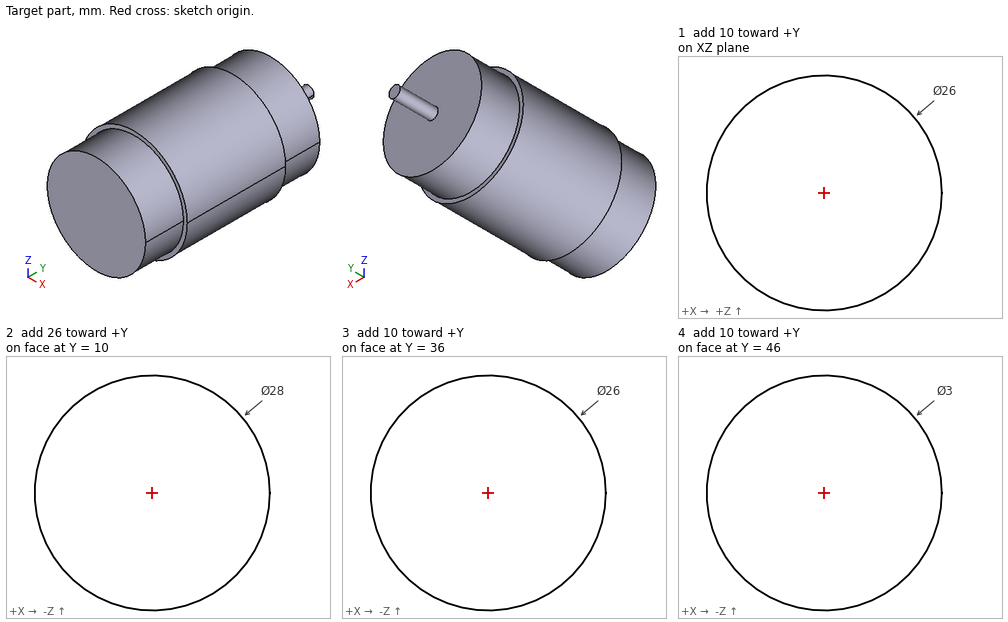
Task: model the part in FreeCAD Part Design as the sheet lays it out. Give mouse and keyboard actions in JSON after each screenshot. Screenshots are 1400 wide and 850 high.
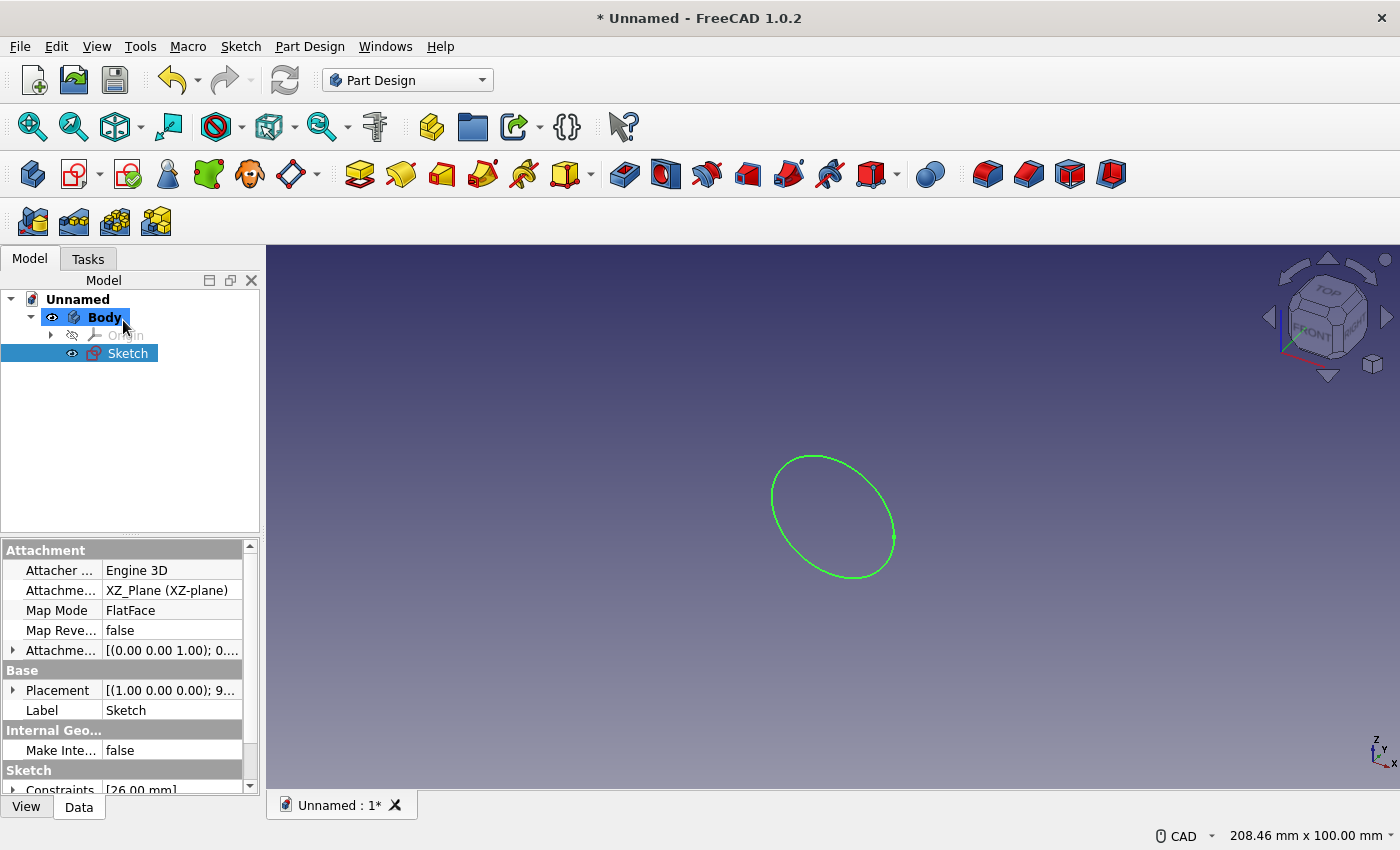
{"action": "left_click", "coordinate": [360, 174]}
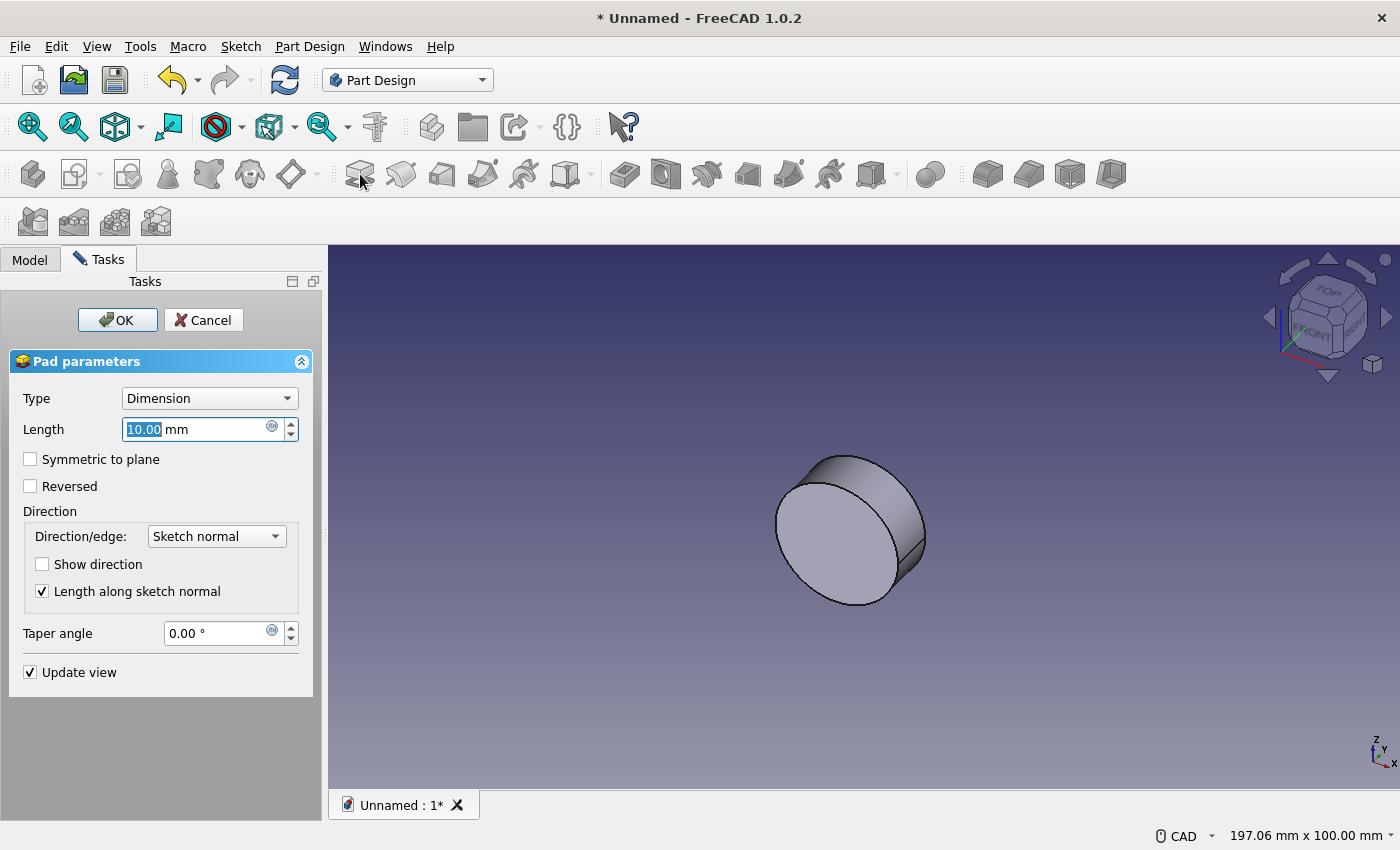
{"action": "type", "text": "10"}
{"action": "key", "text": "Tab"}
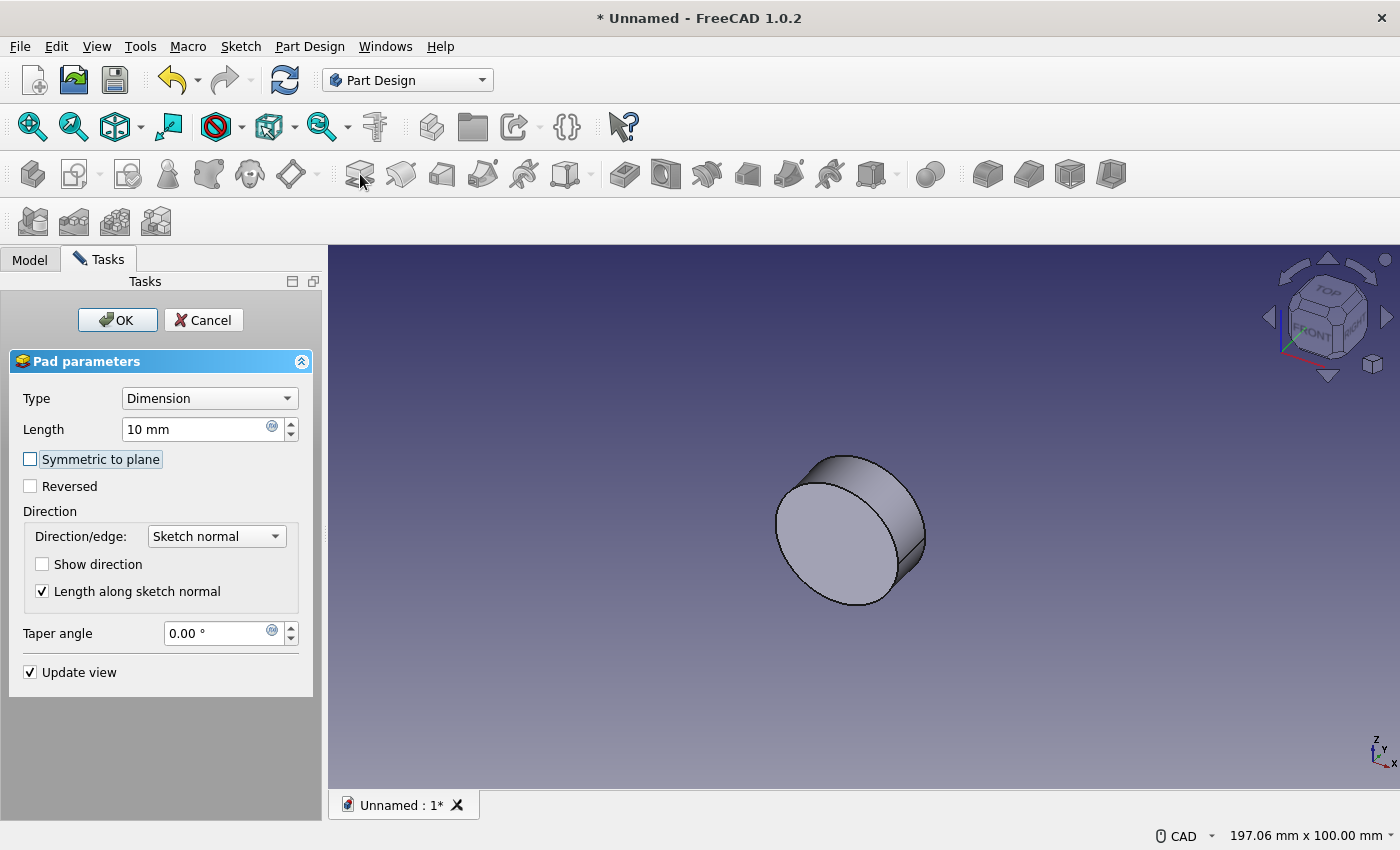
{"action": "left_click", "coordinate": [31, 486]}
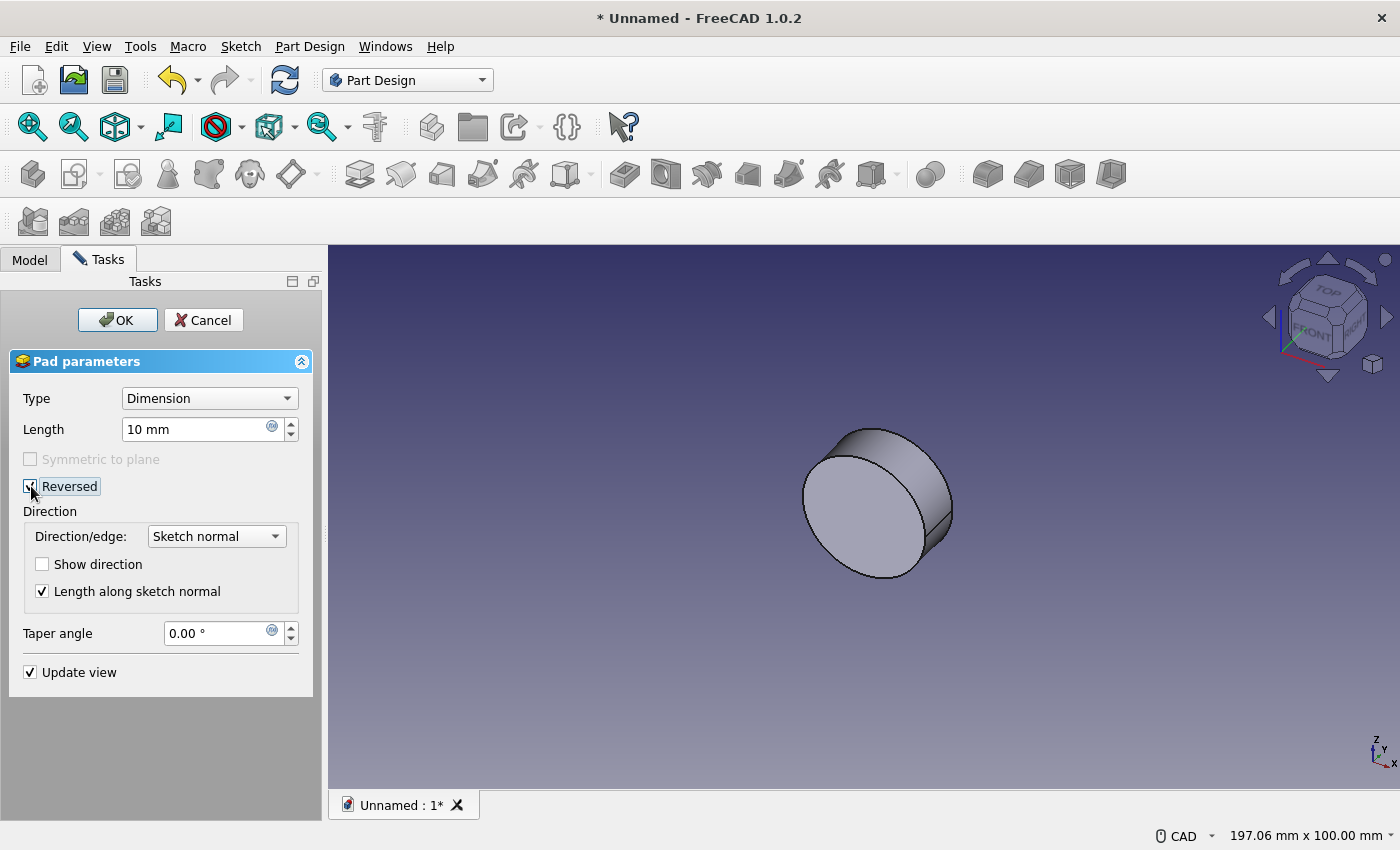
{"action": "left_click", "coordinate": [118, 320]}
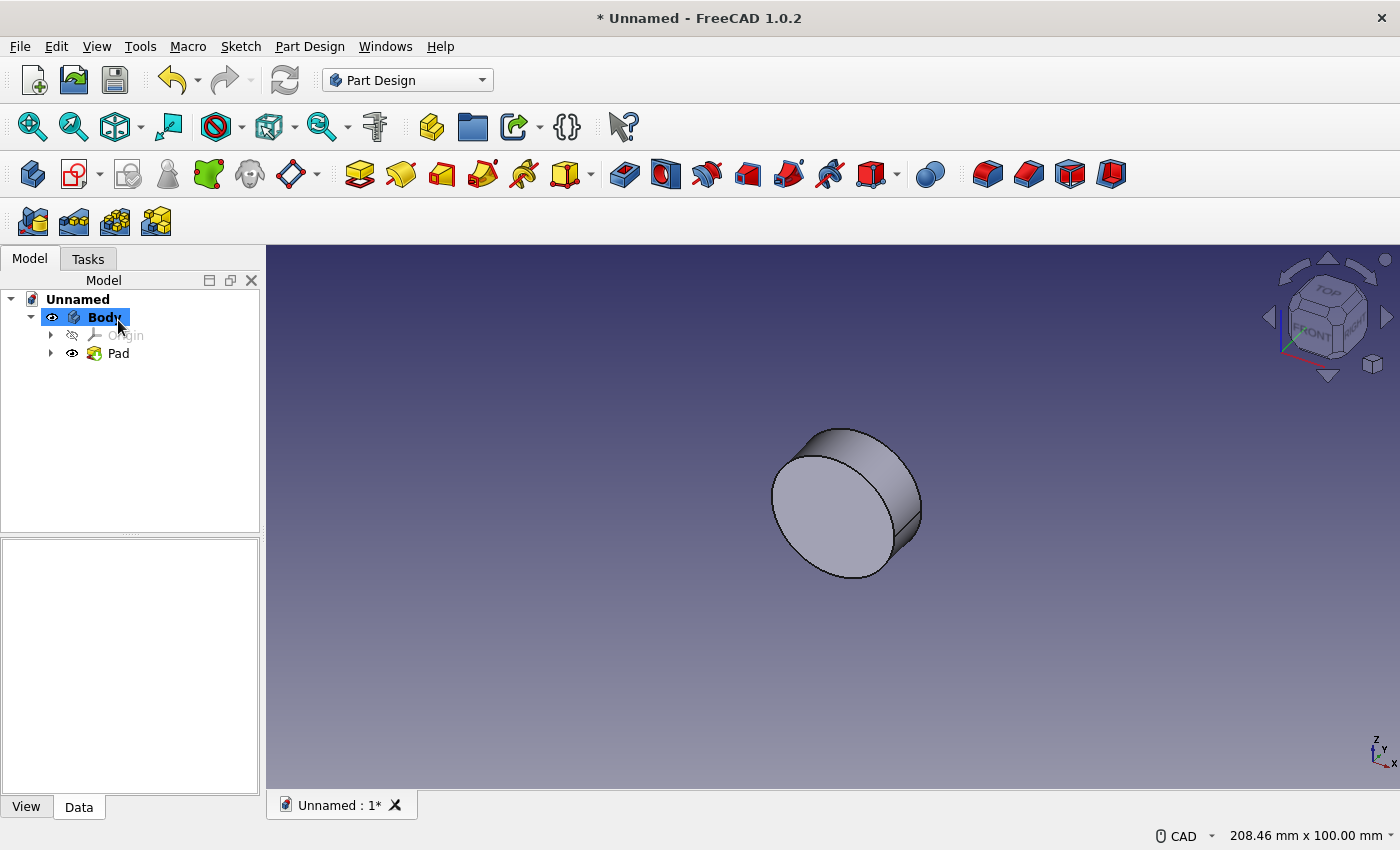
{"action": "left_click", "coordinate": [33, 128]}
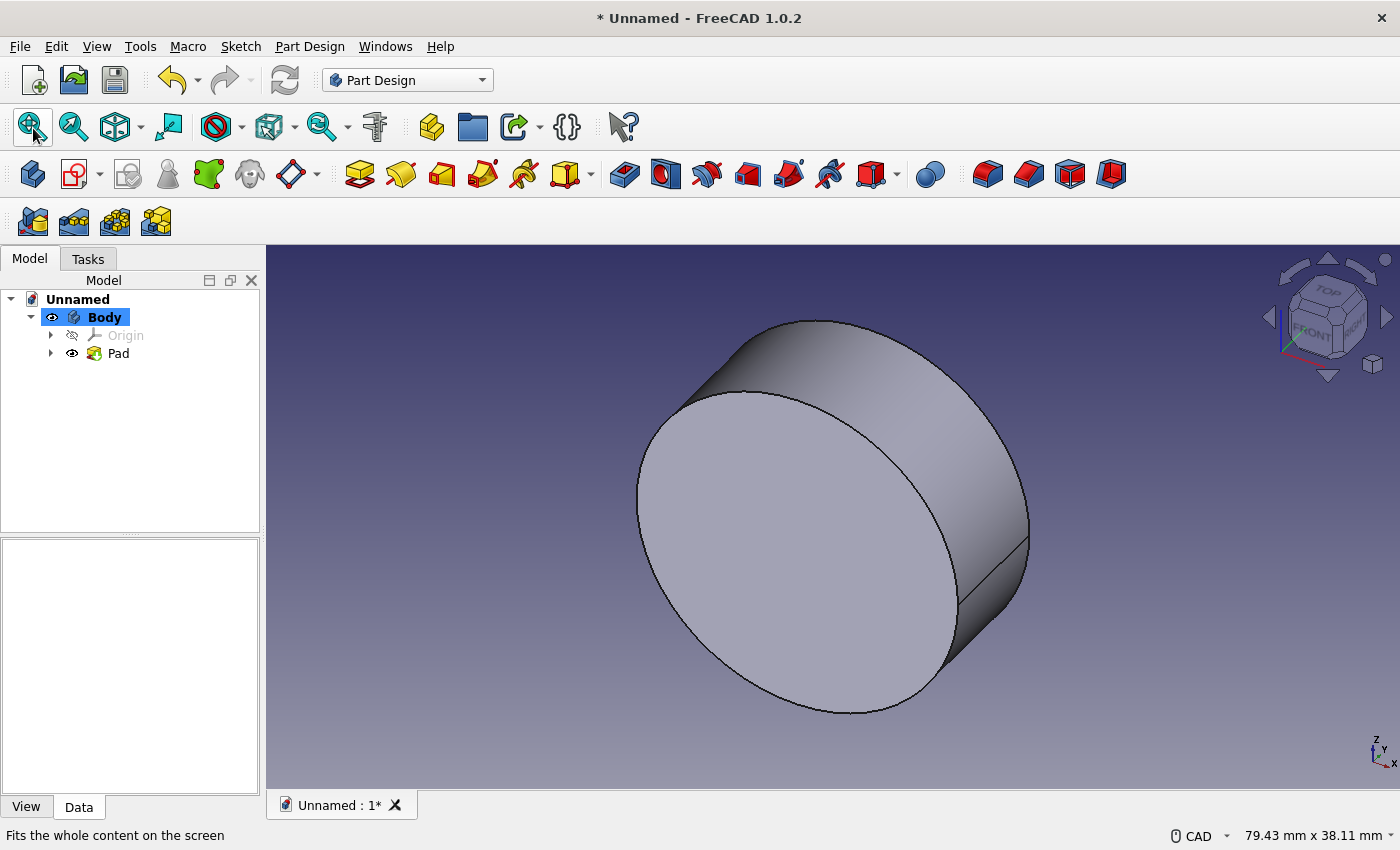
{"action": "key", "text": "4"}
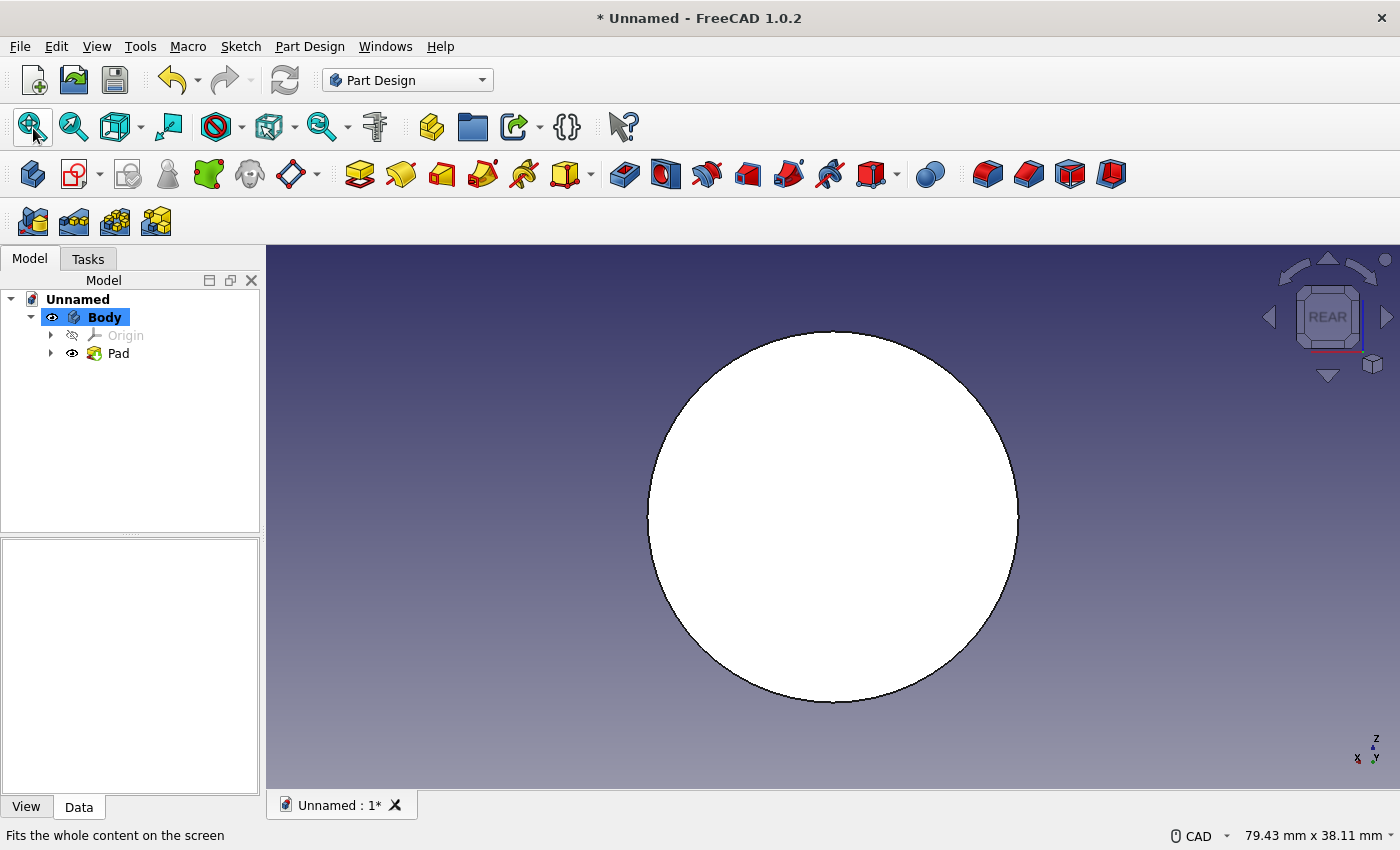
{"action": "left_click", "coordinate": [833, 516]}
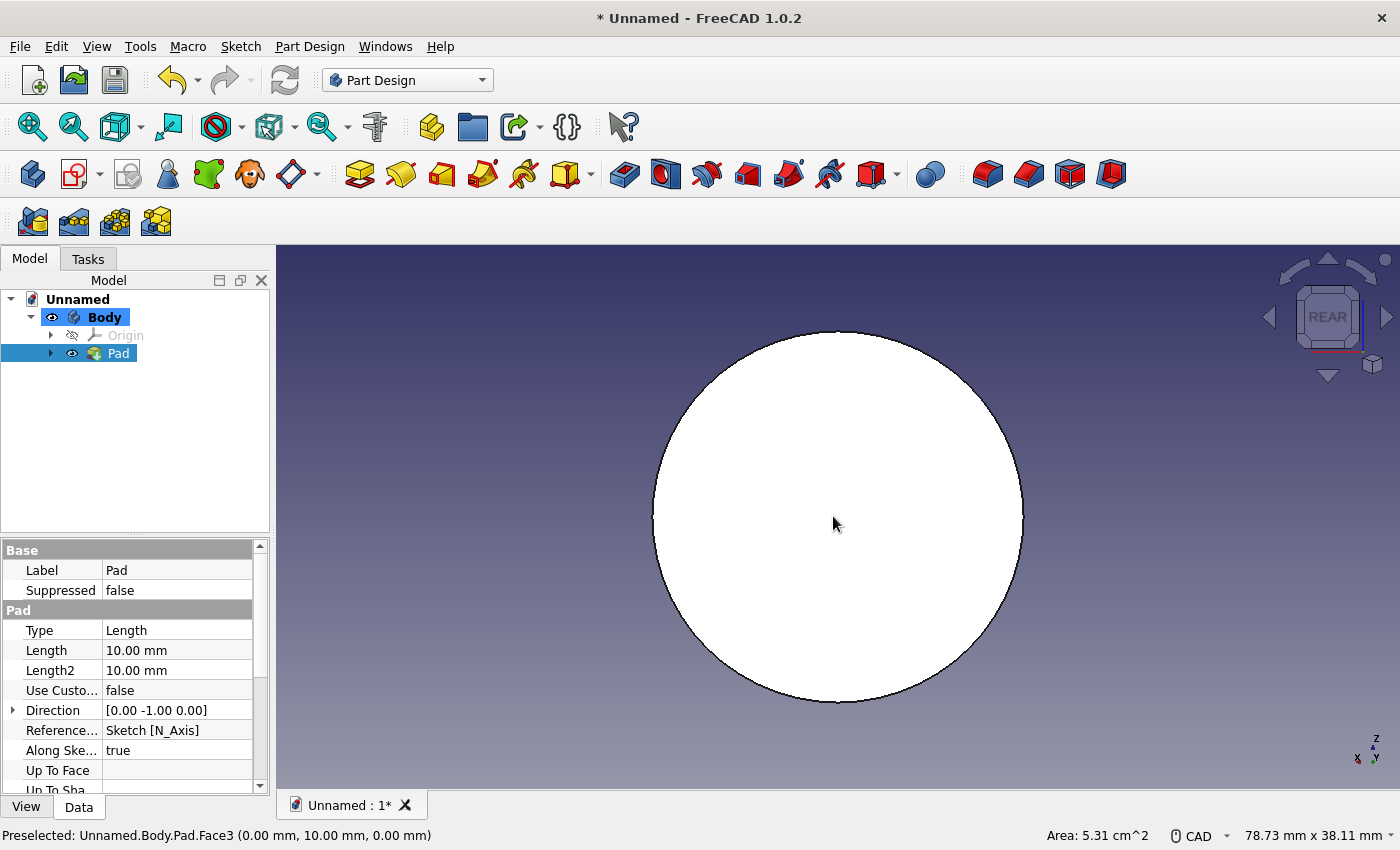
{"action": "left_click", "coordinate": [74, 174]}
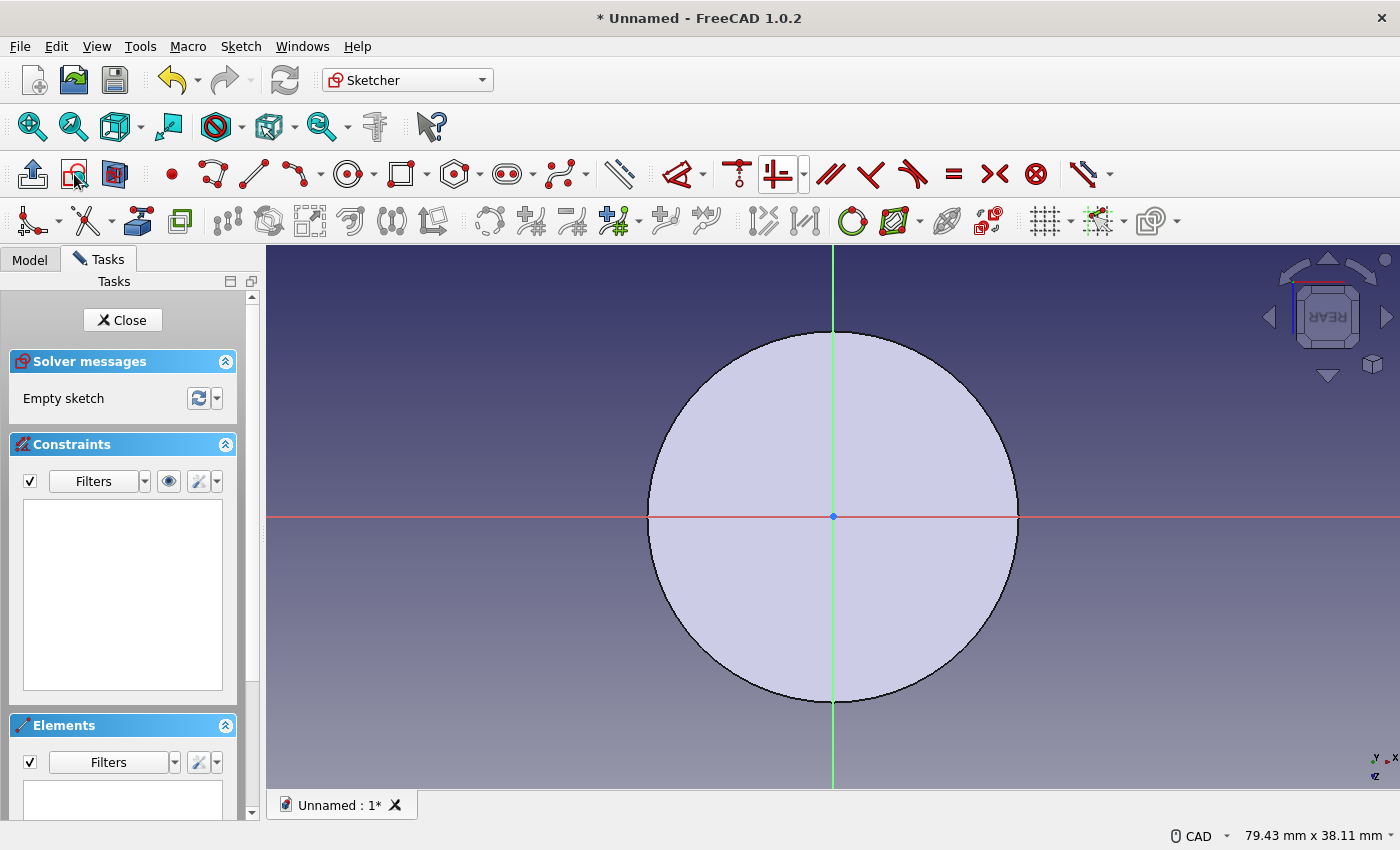
{"action": "key", "text": "g c"}